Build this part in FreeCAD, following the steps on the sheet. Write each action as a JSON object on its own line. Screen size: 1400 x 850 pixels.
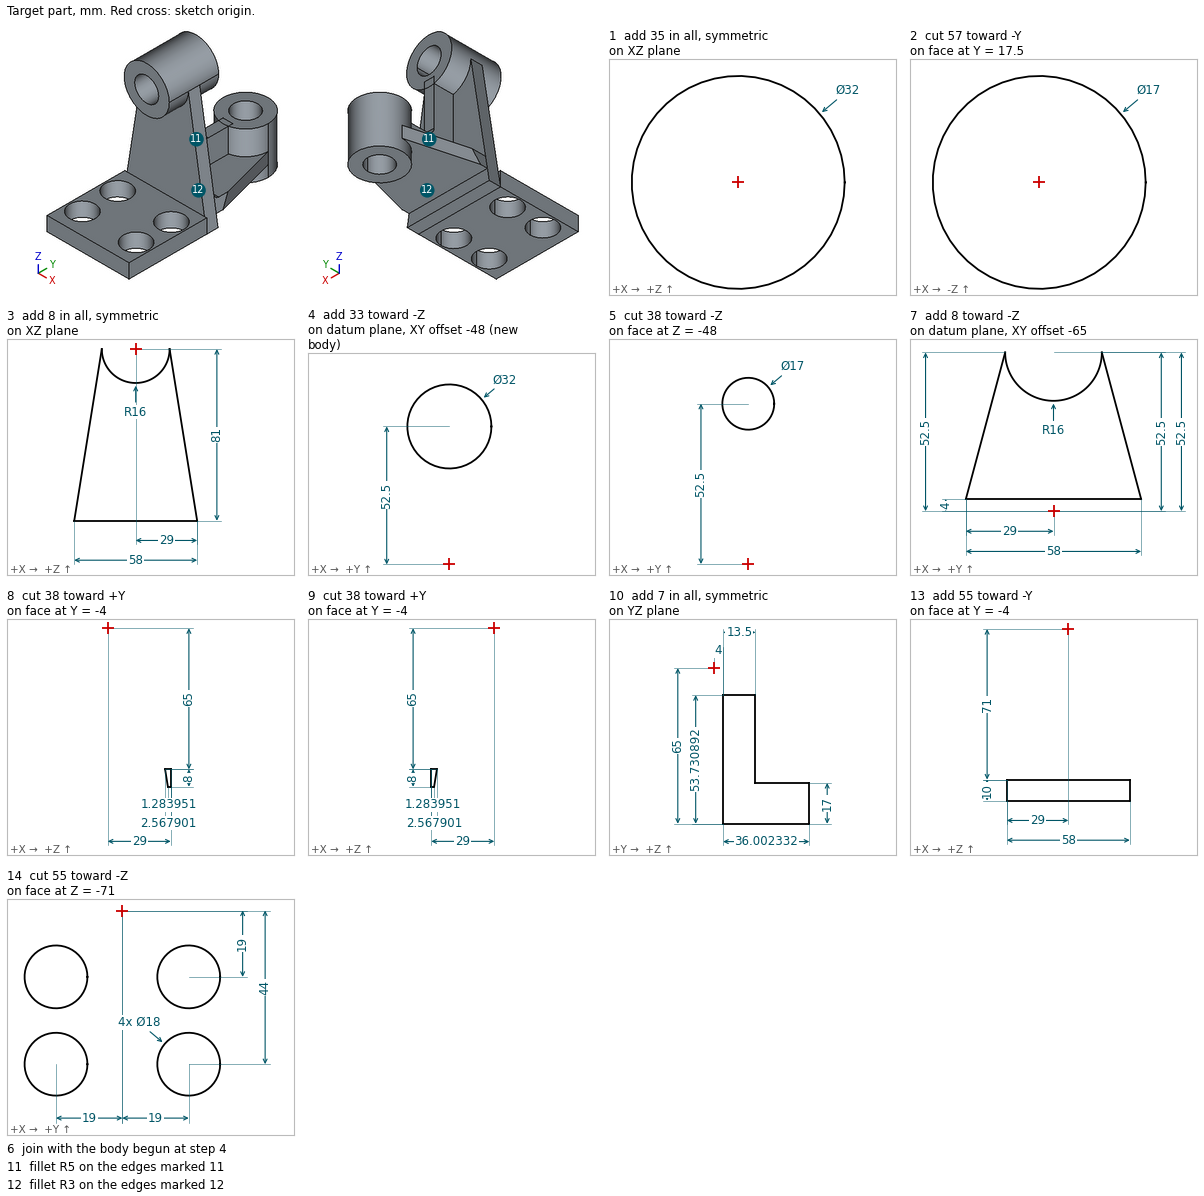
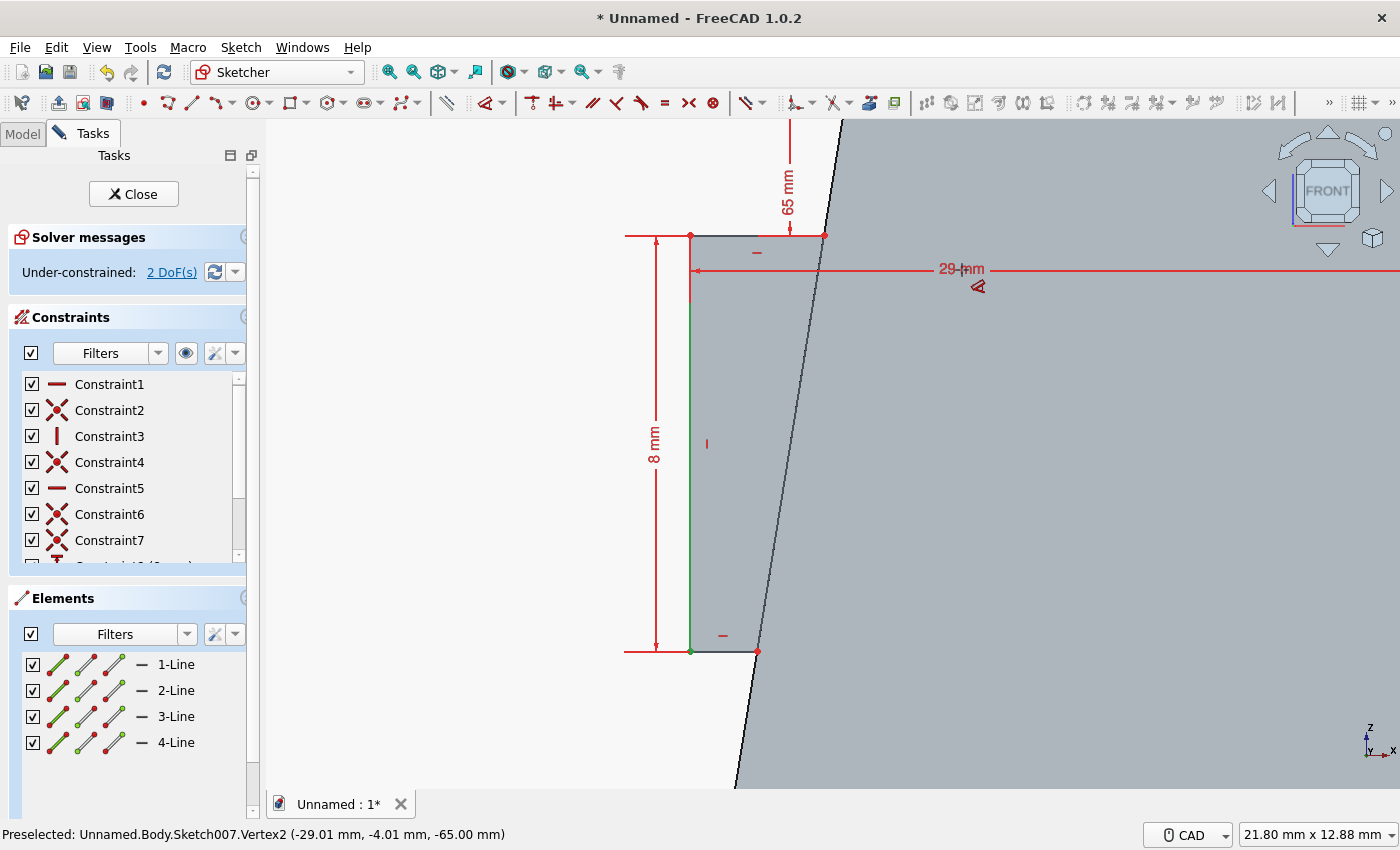
{"action": "left_click", "coordinate": [784, 236]}
{"action": "left_click", "coordinate": [710, 202]}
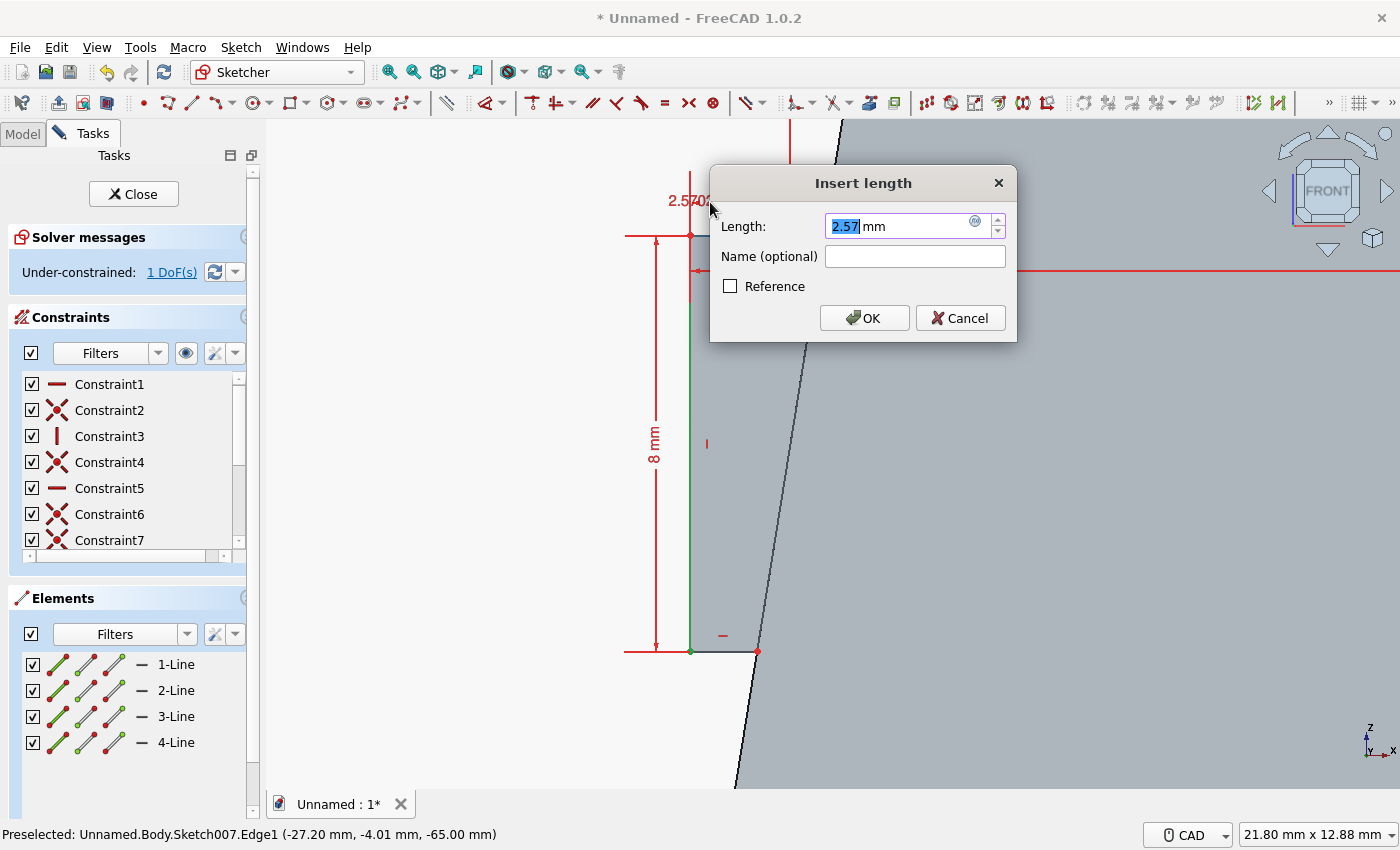
{"action": "type", "text": "2.567901"}
{"action": "key", "text": "Return"}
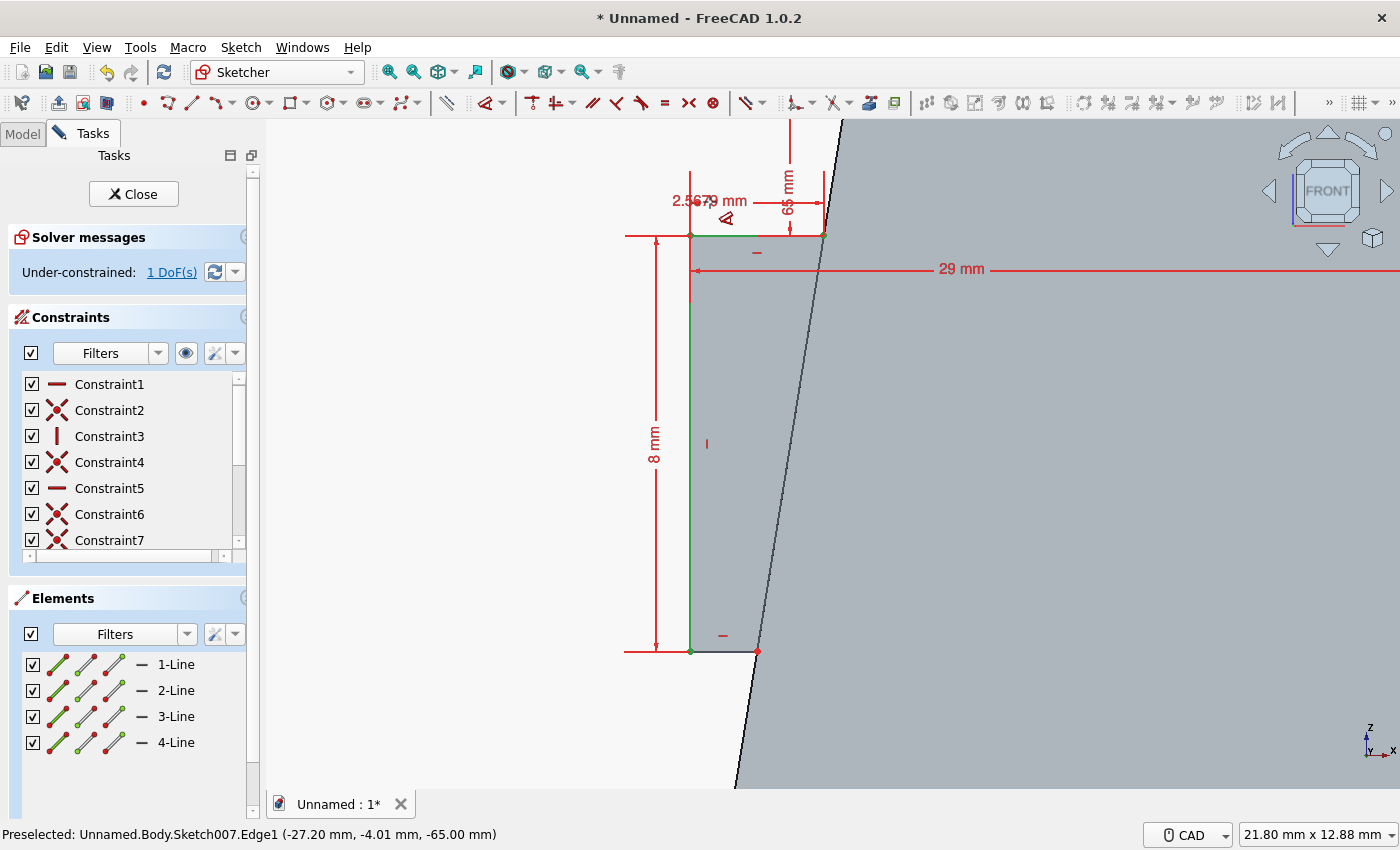
{"action": "left_click", "coordinate": [710, 652]}
{"action": "left_click", "coordinate": [724, 686]}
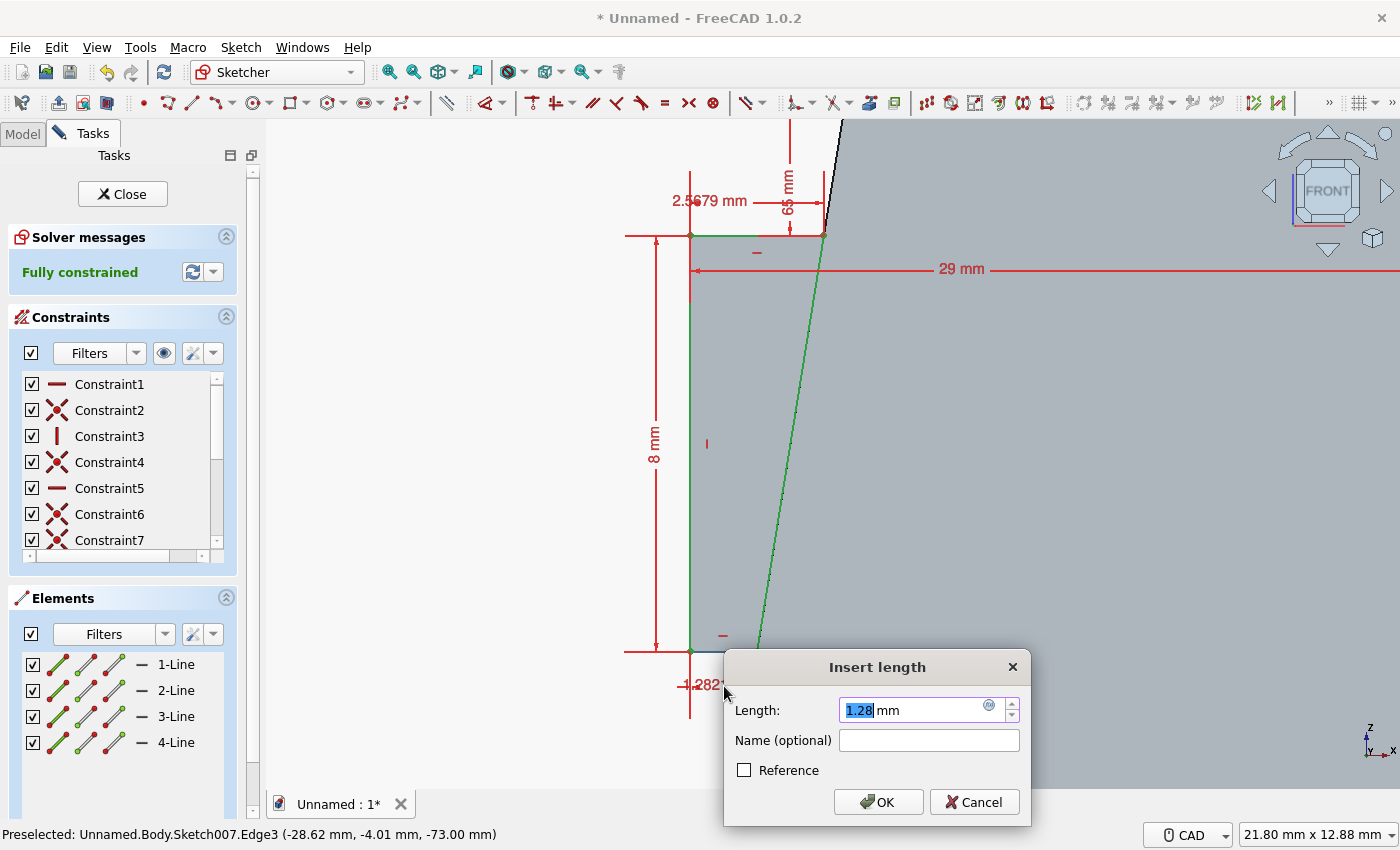
{"action": "type", "text": "1.283951"}
{"action": "key", "text": "Return"}
{"action": "key", "text": "Escape"}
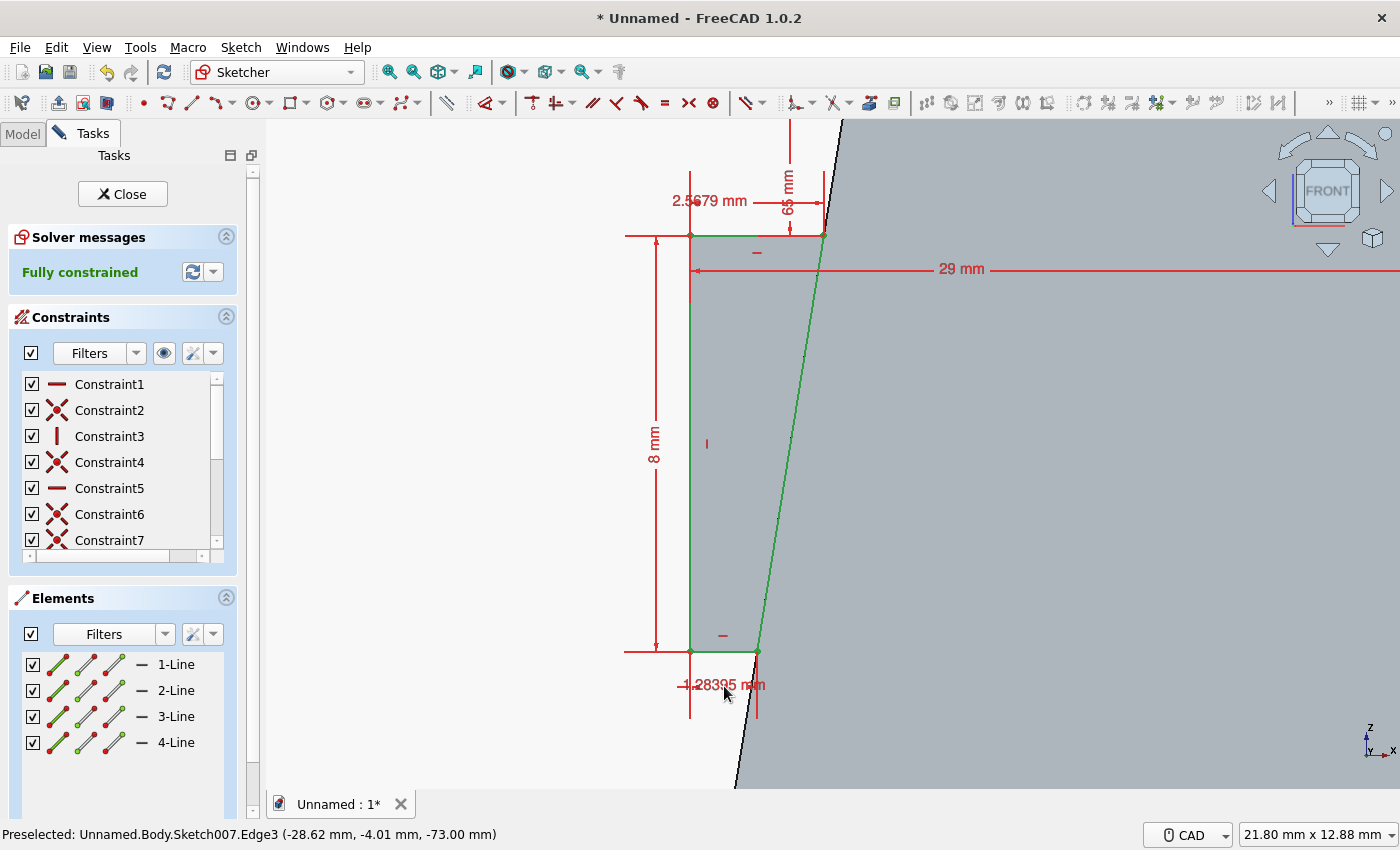
{"action": "left_click", "coordinate": [123, 194]}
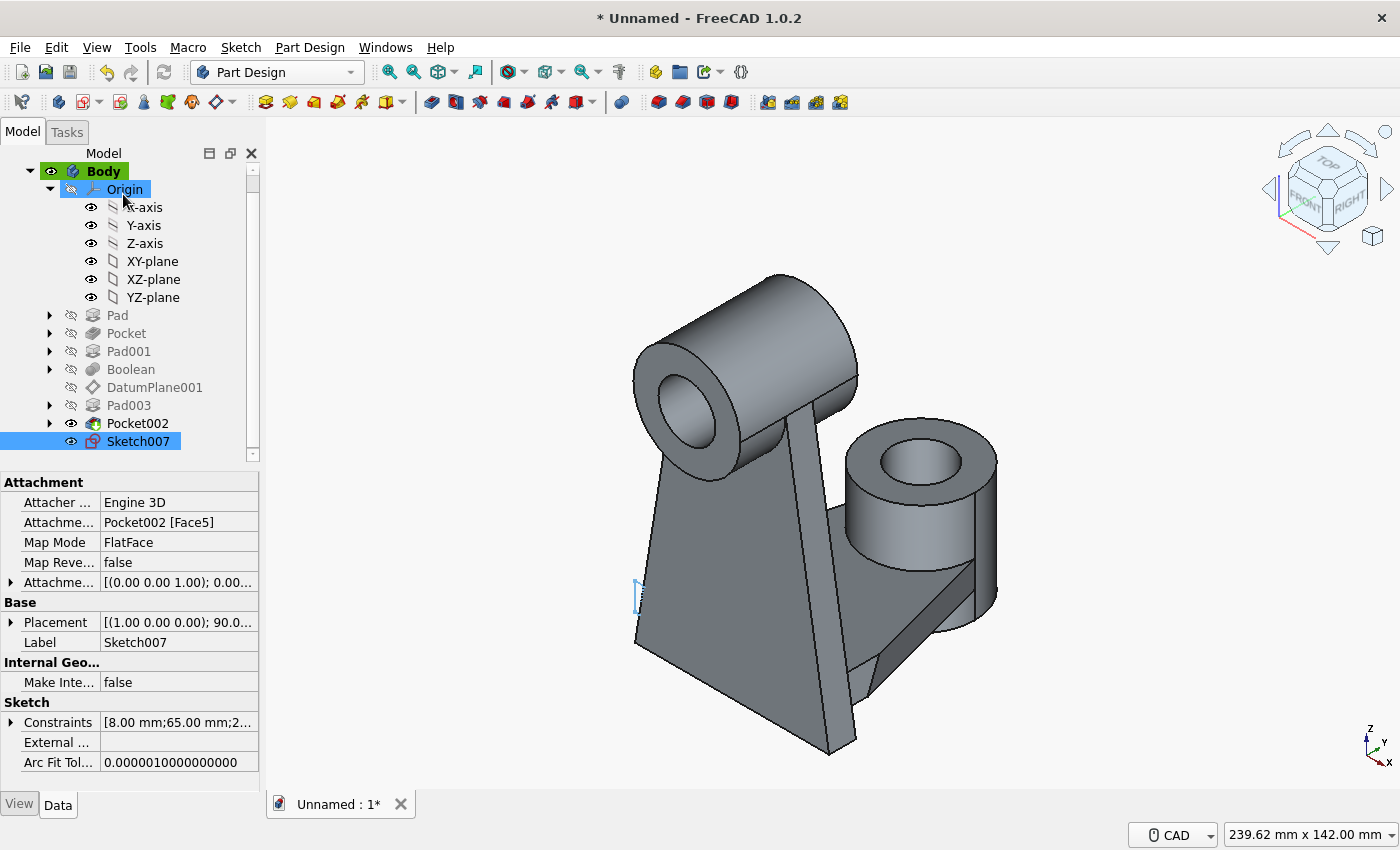
{"action": "left_click", "coordinate": [432, 102]}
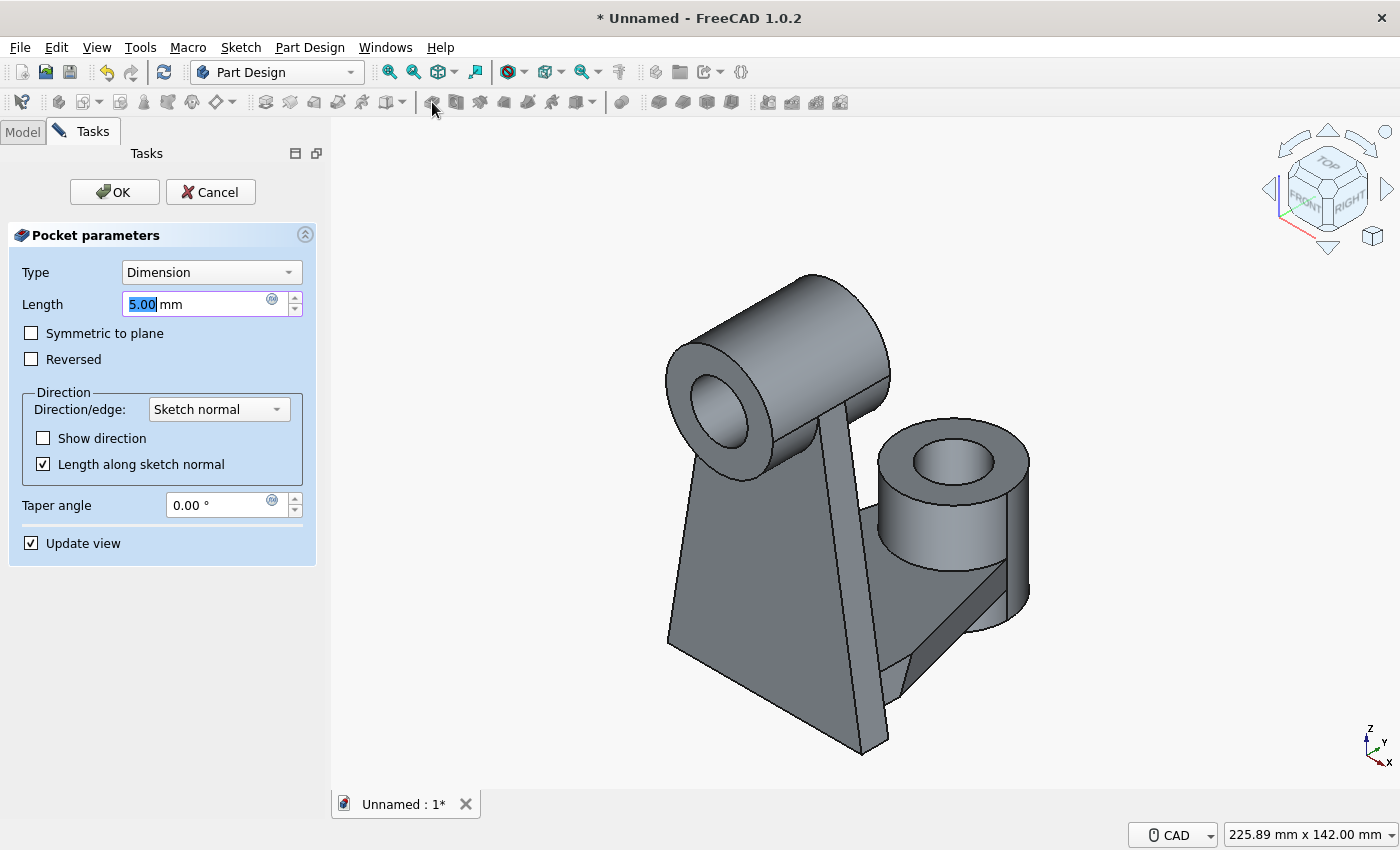
{"action": "type", "text": "38"}
{"action": "key", "text": "Tab"}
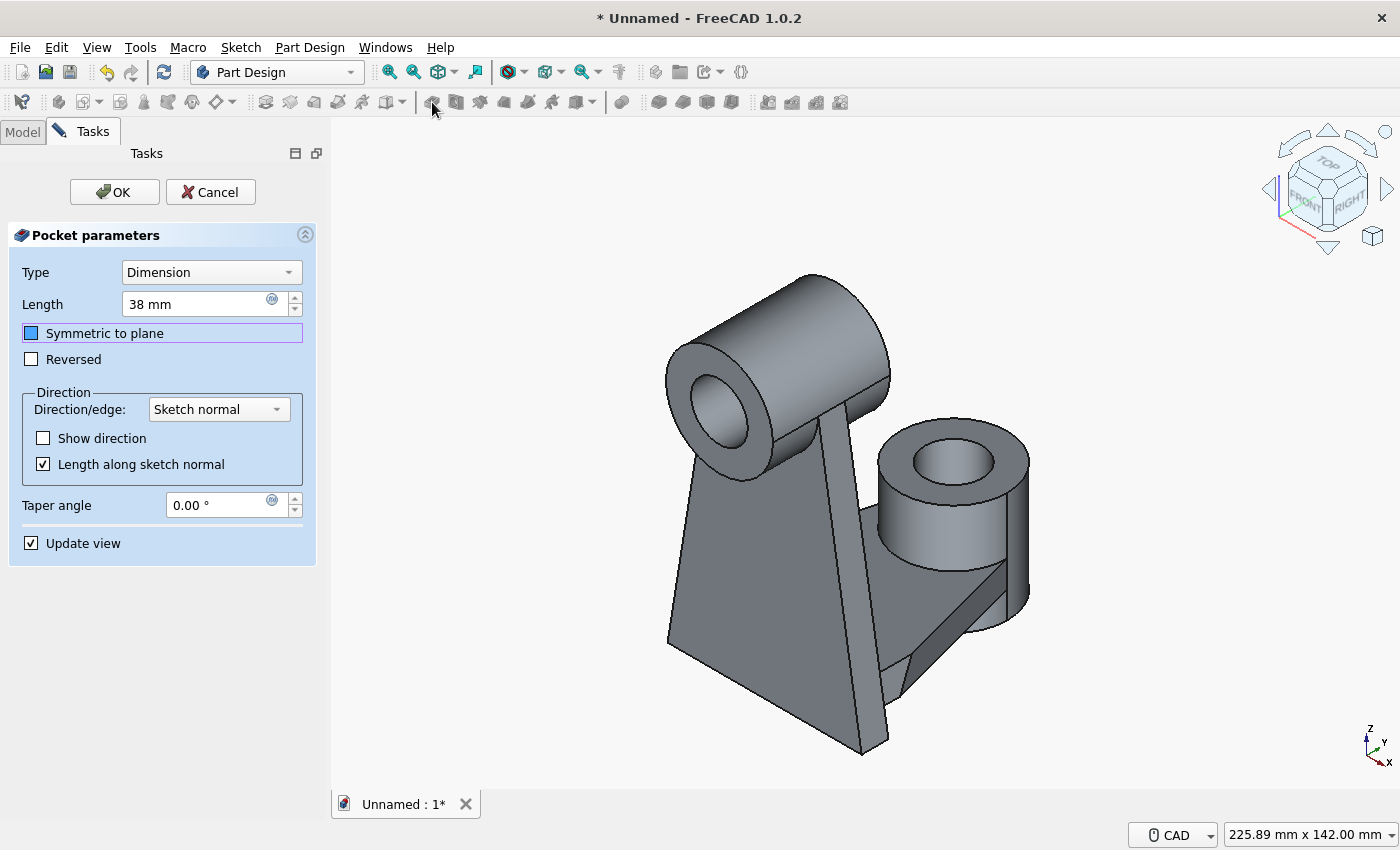
{"action": "left_click", "coordinate": [115, 192]}